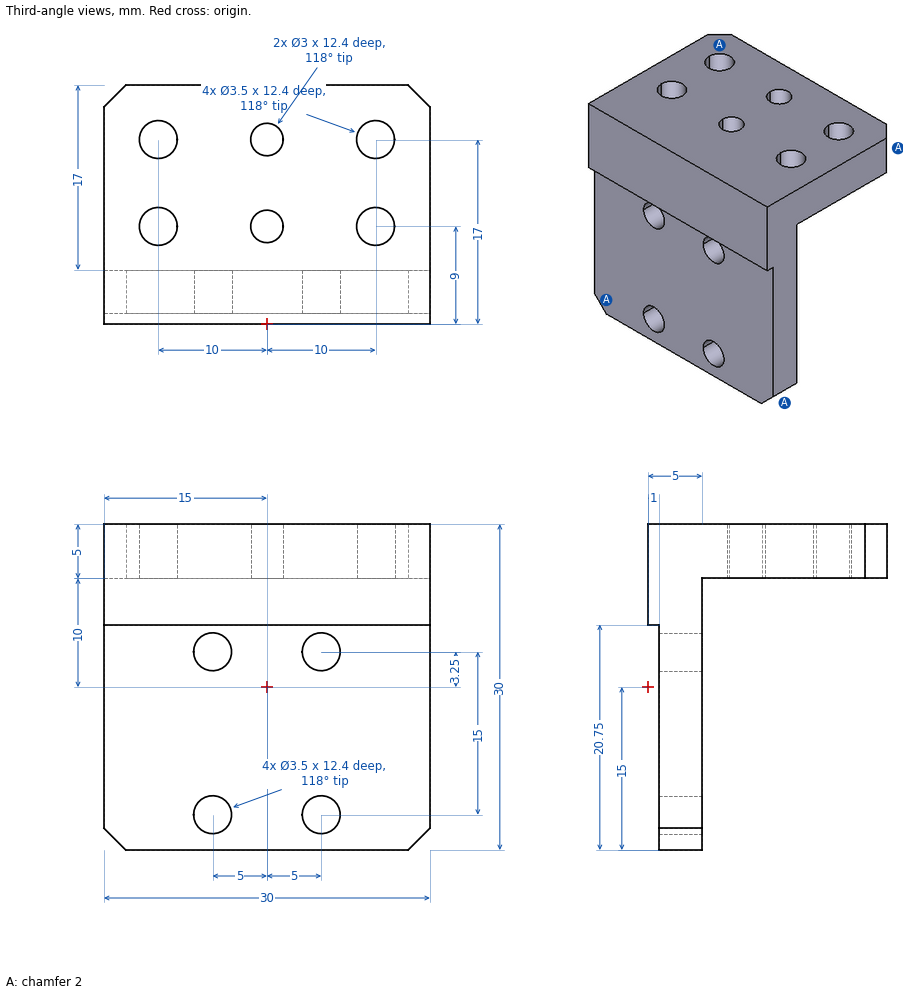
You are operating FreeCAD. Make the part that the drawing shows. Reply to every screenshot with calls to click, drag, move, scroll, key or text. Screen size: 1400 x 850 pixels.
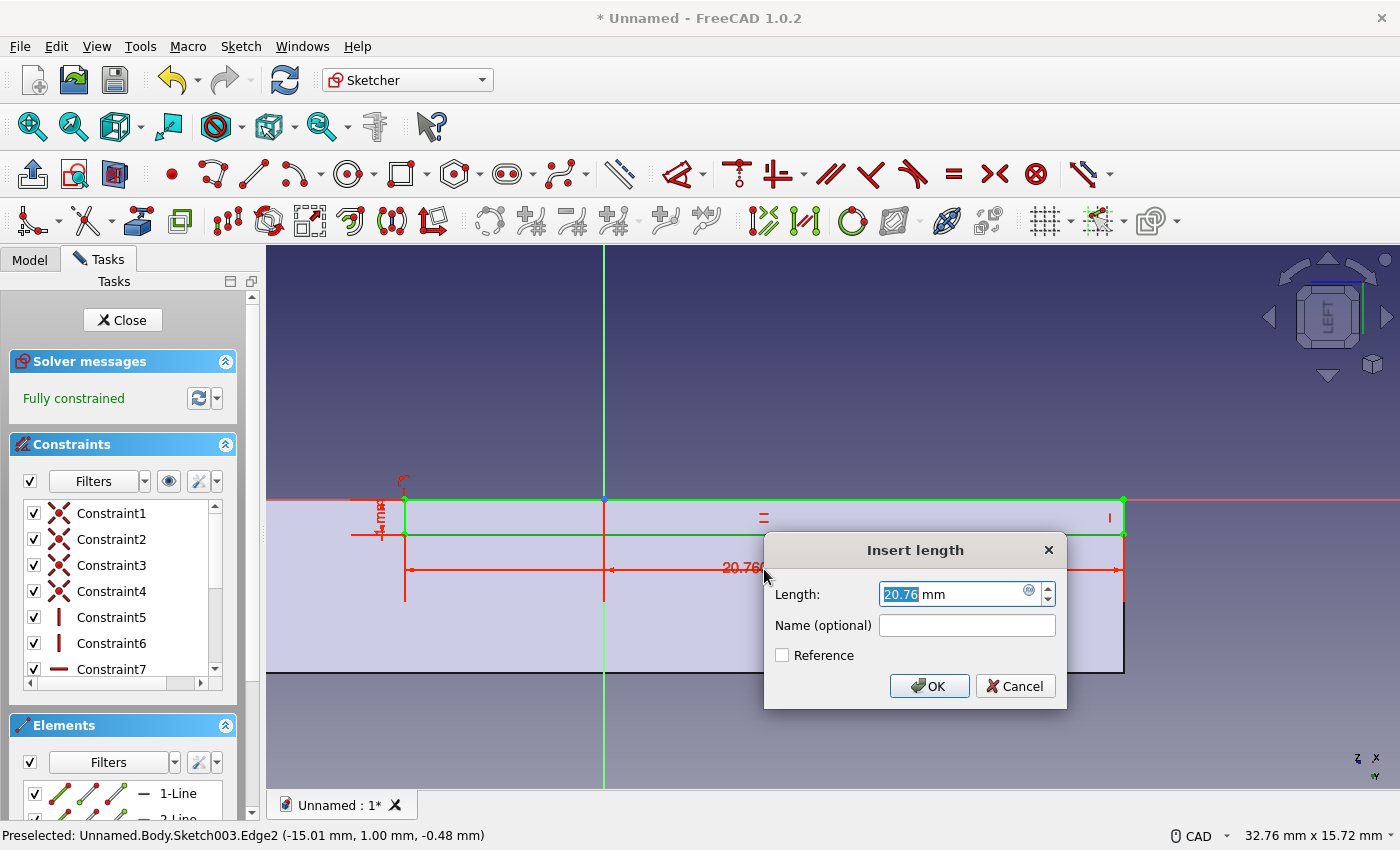
text(20.75)
key(Return)
key(Escape)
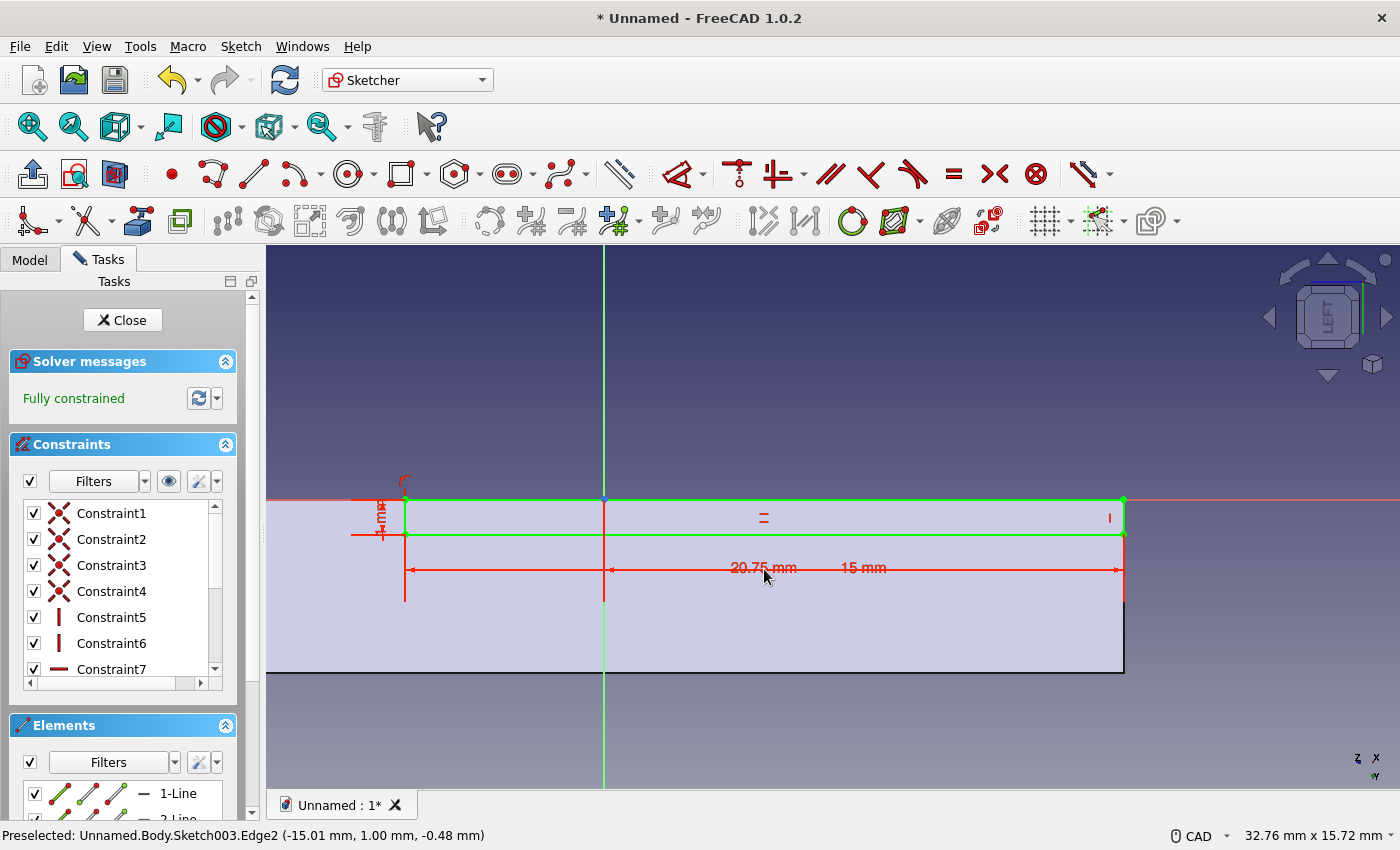
click(123, 320)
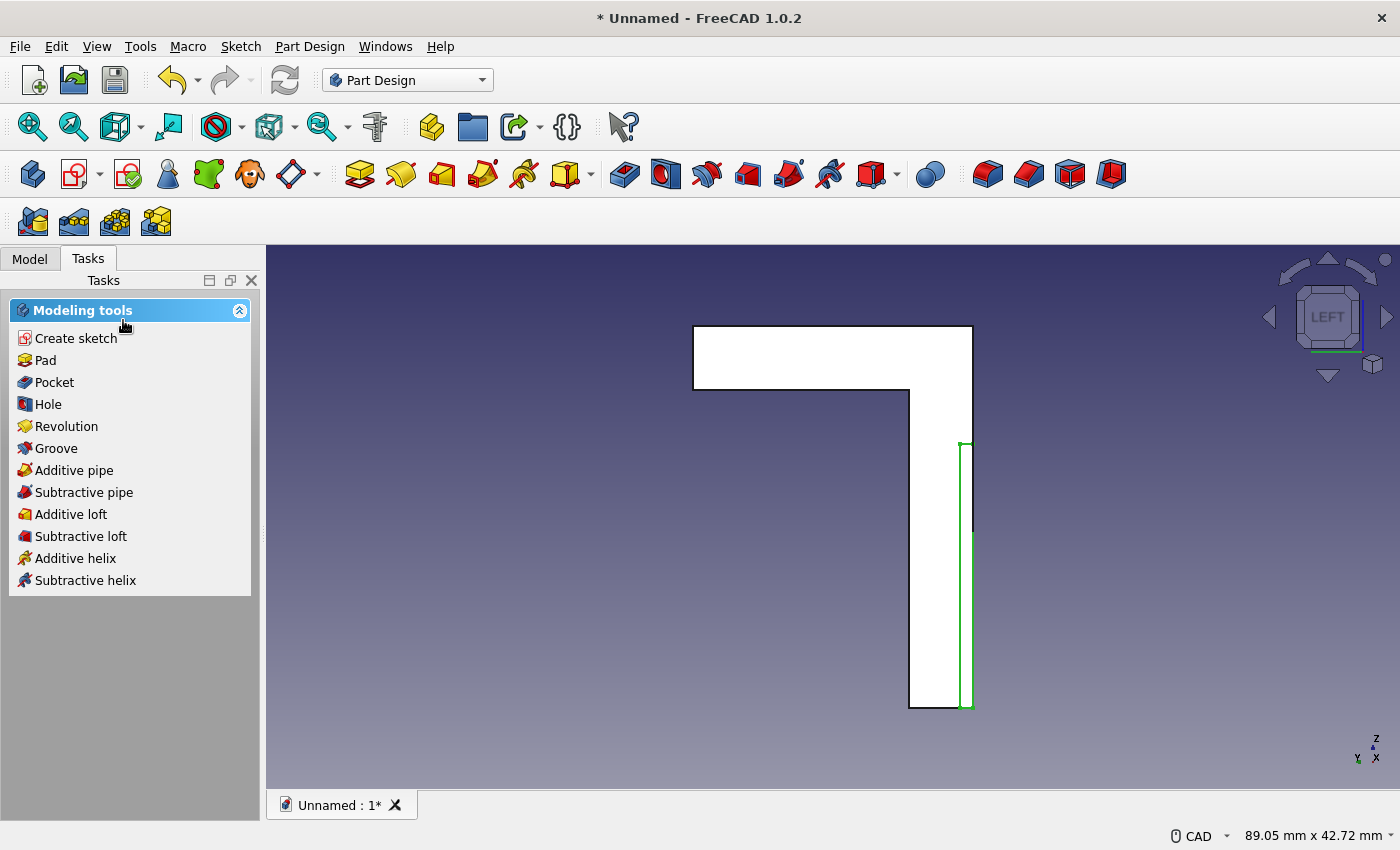
click(625, 174)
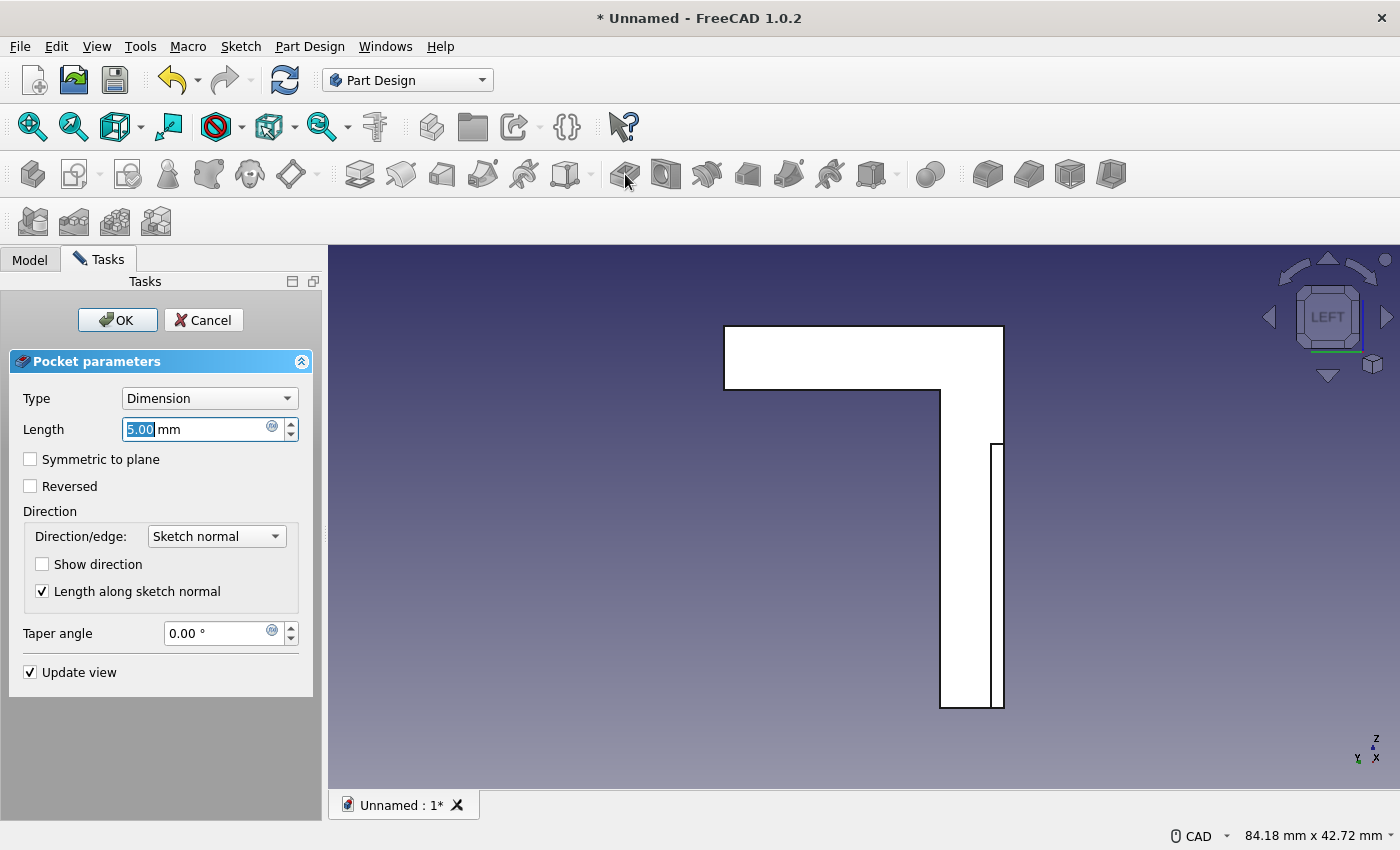
click(210, 398)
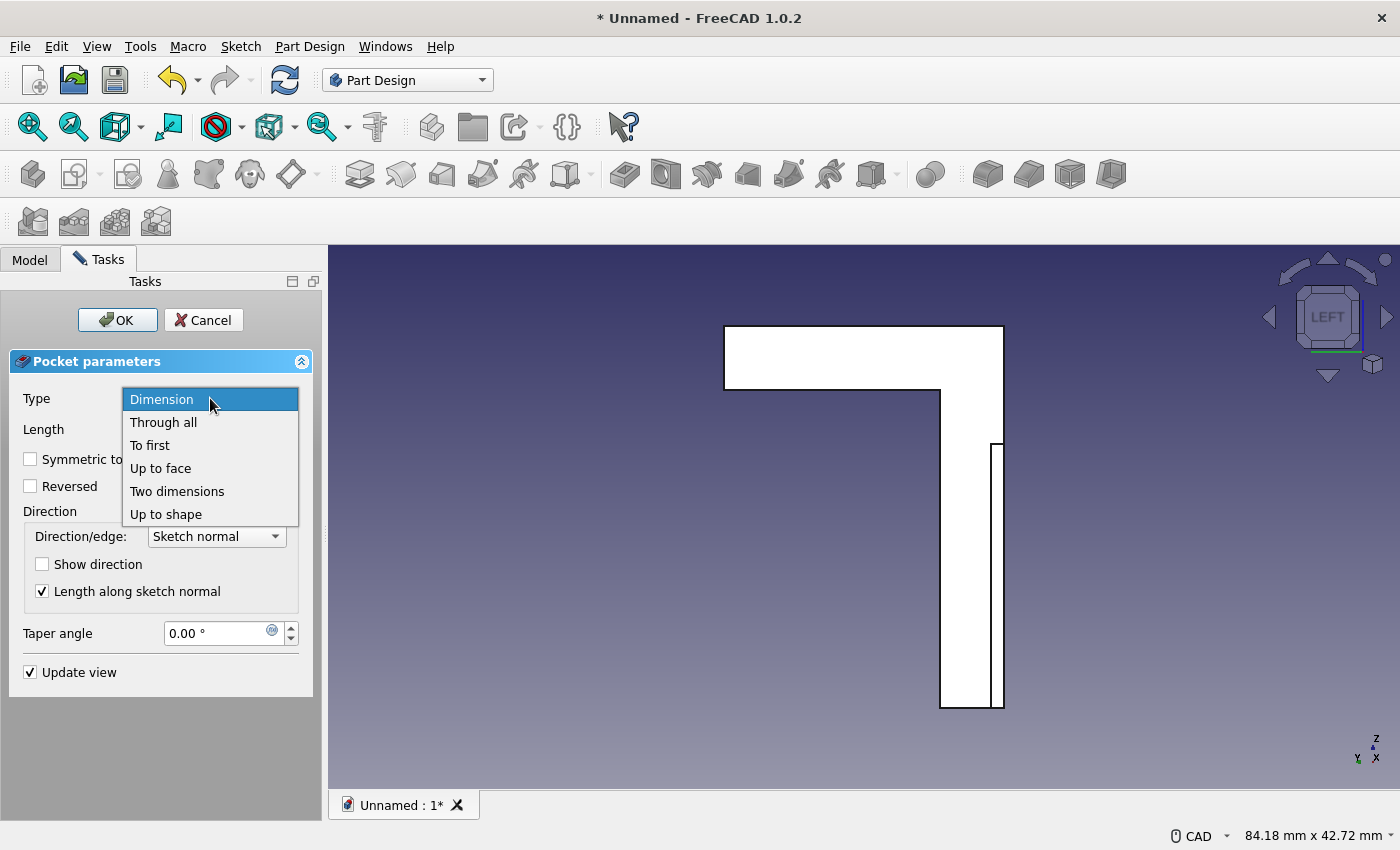
click(208, 422)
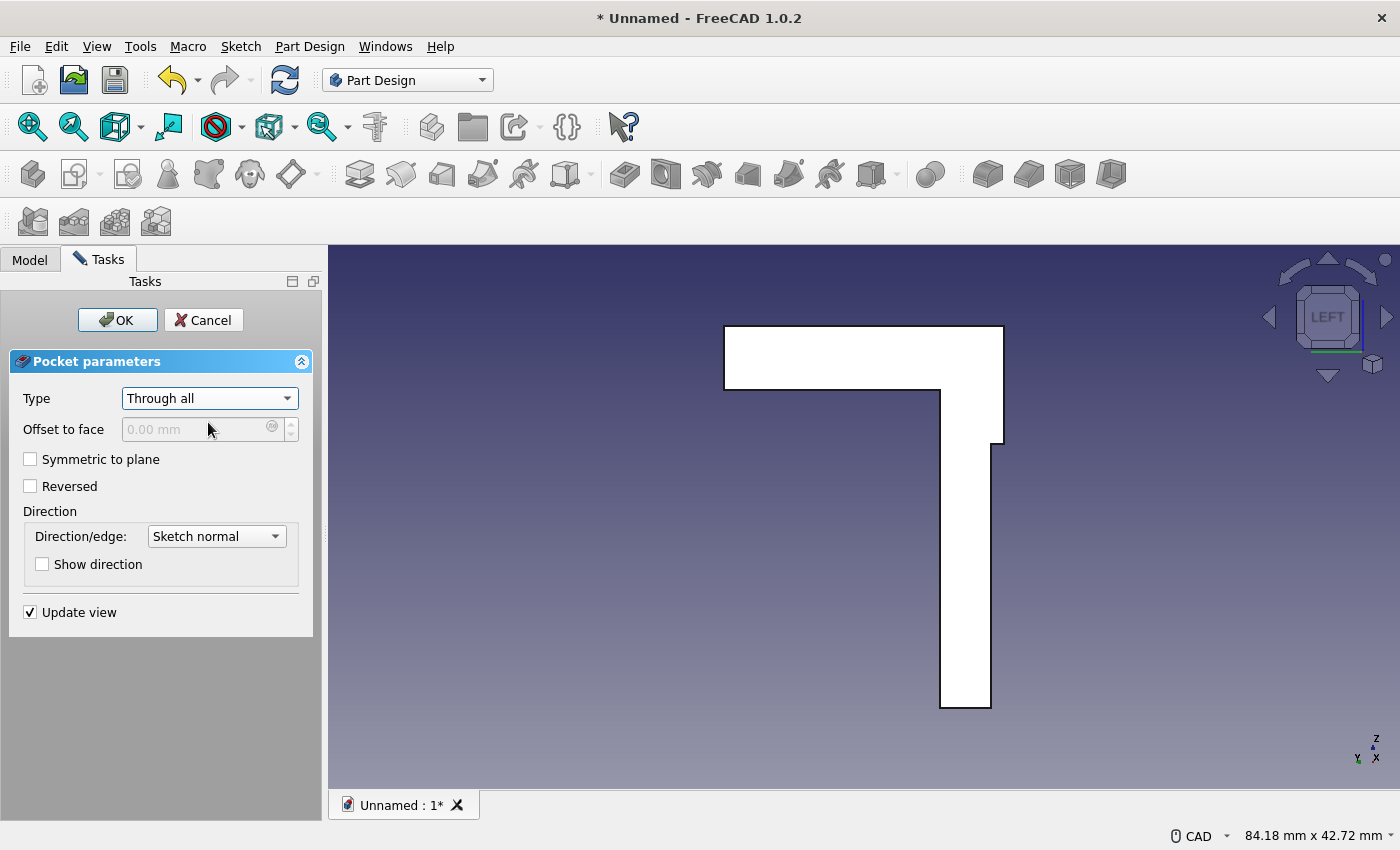
click(118, 320)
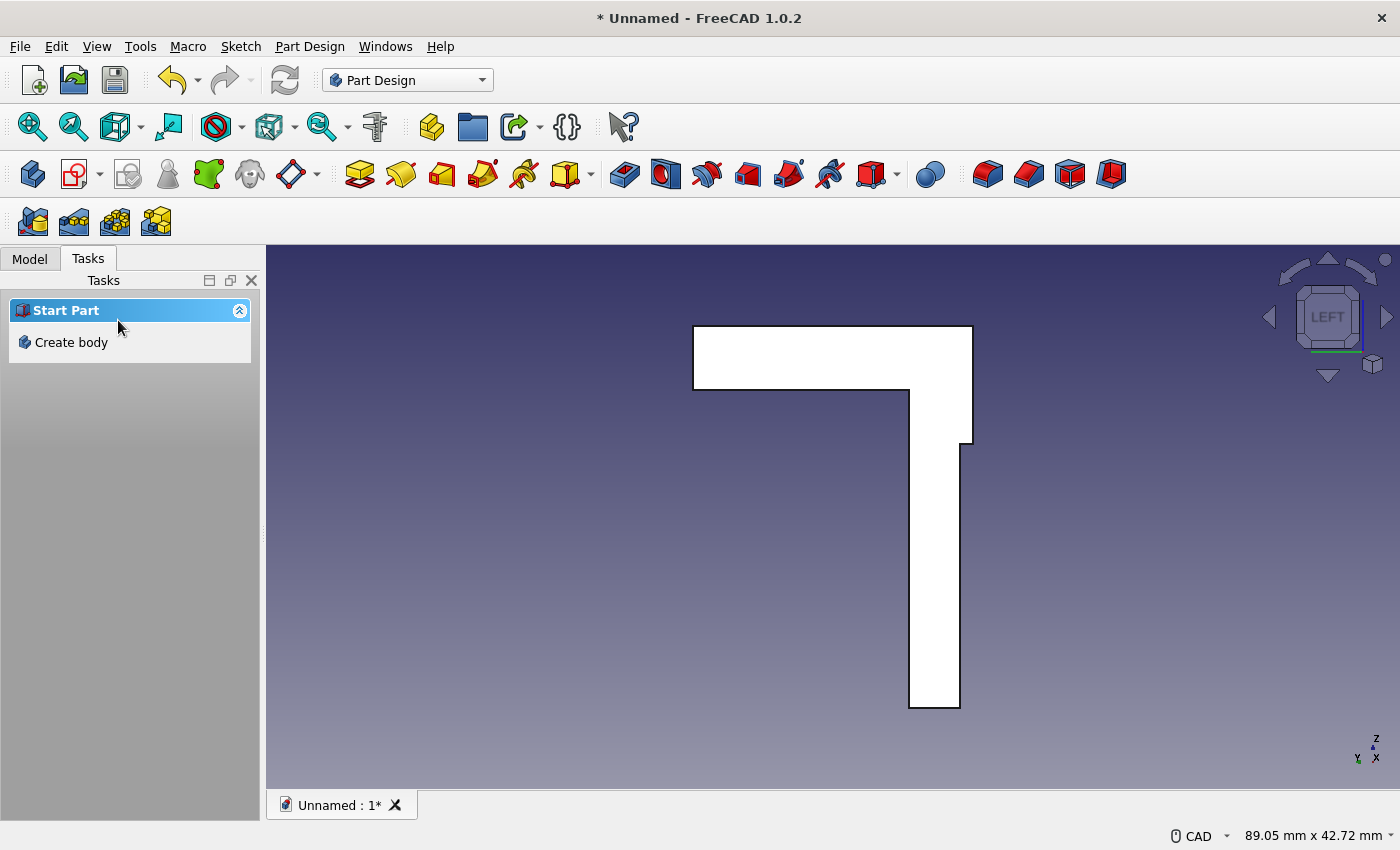
click(693, 357)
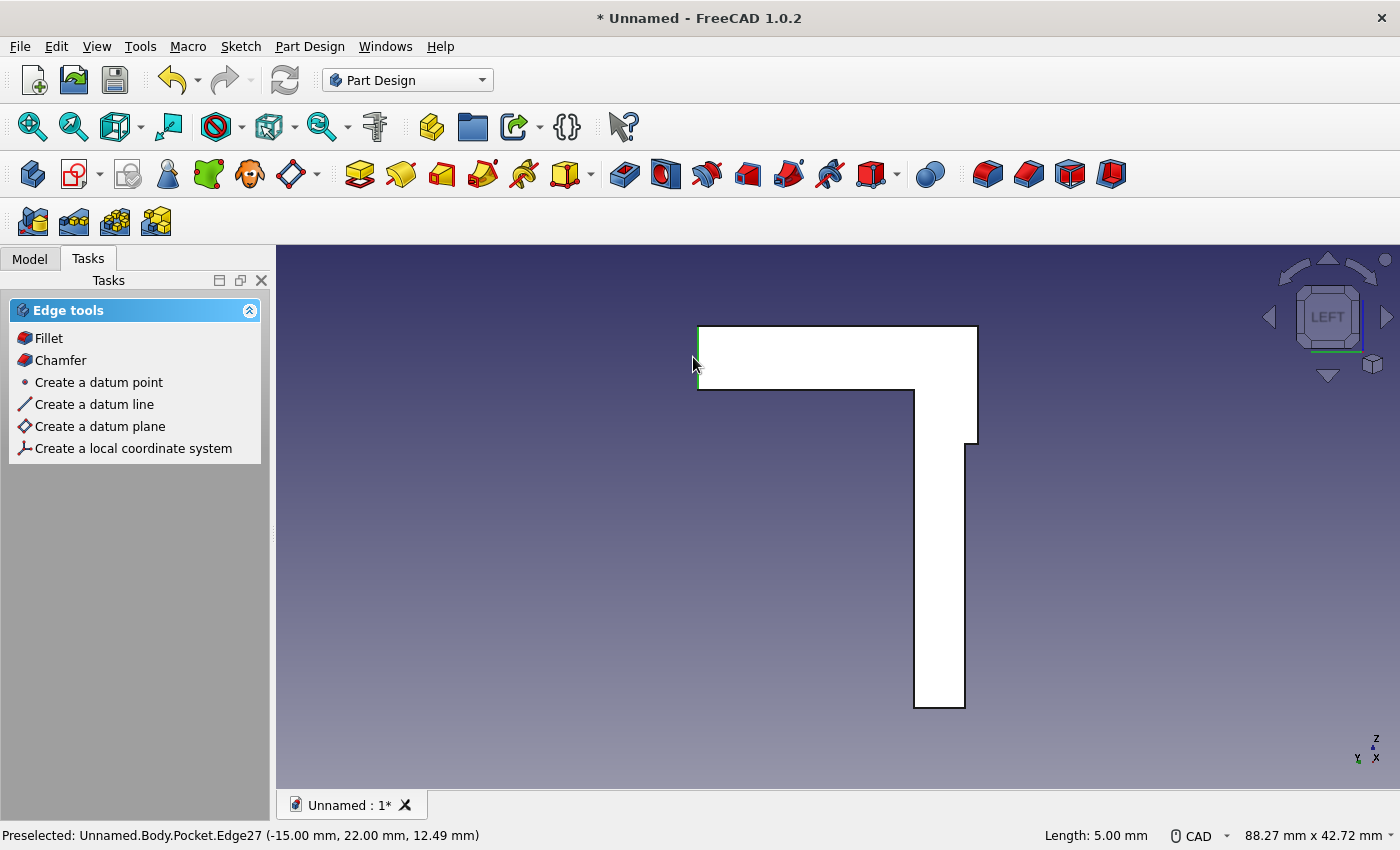
click(940, 707, ctrl)